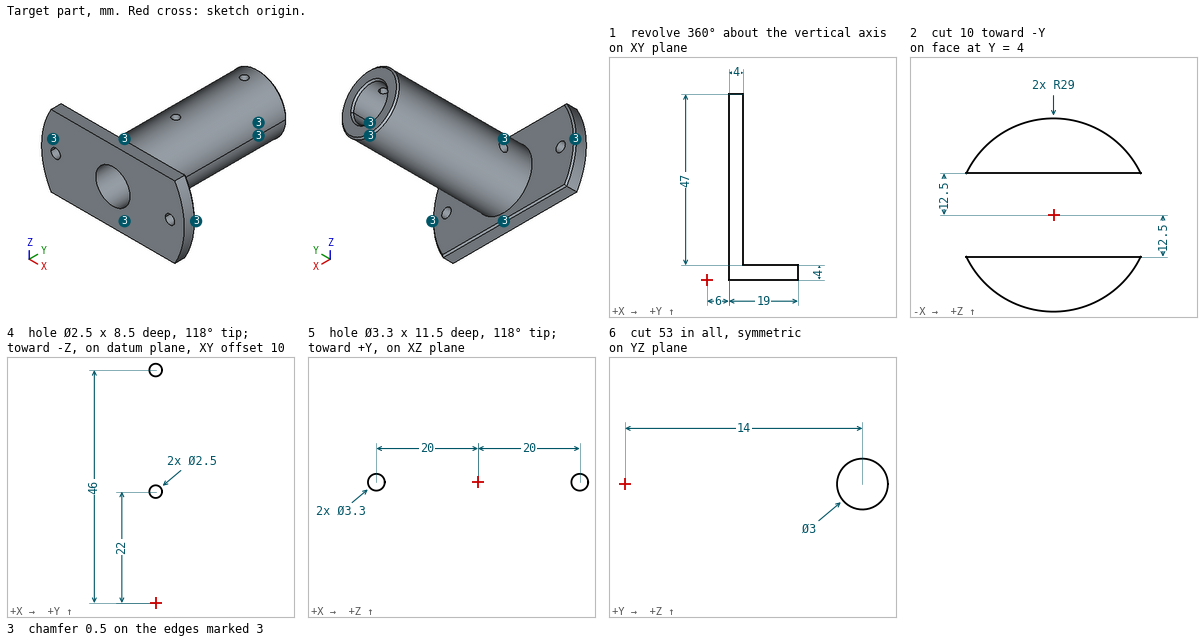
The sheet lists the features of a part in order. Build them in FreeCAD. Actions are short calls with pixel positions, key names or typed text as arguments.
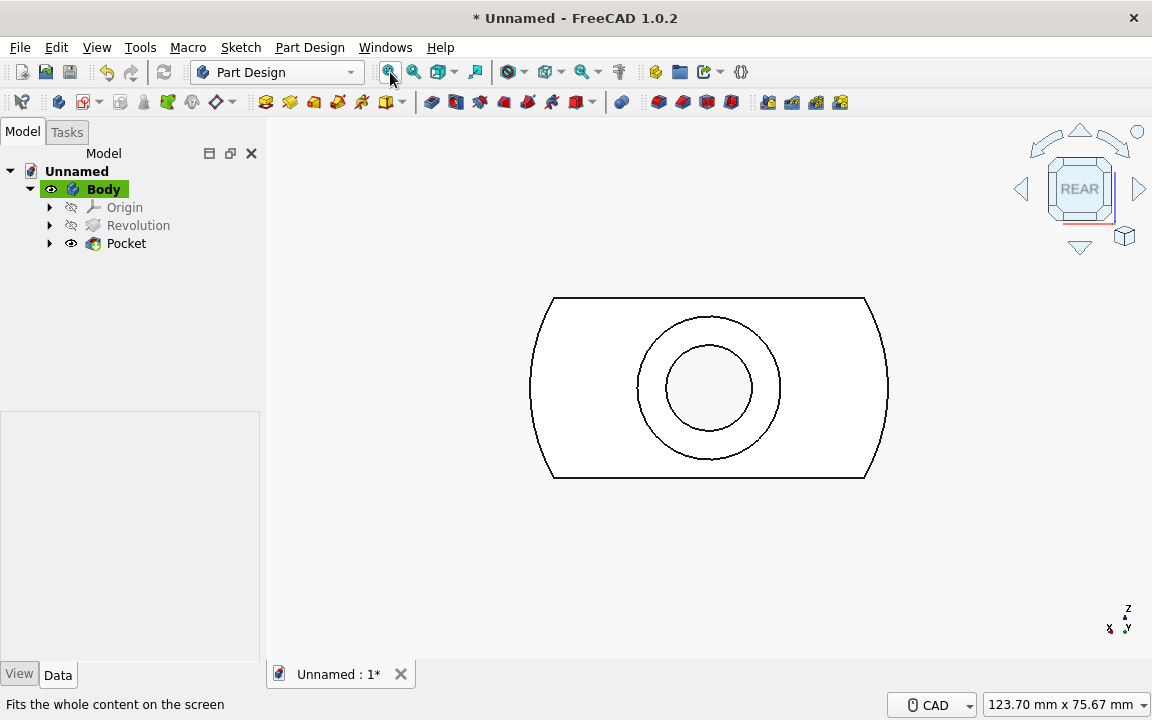
click(888, 387)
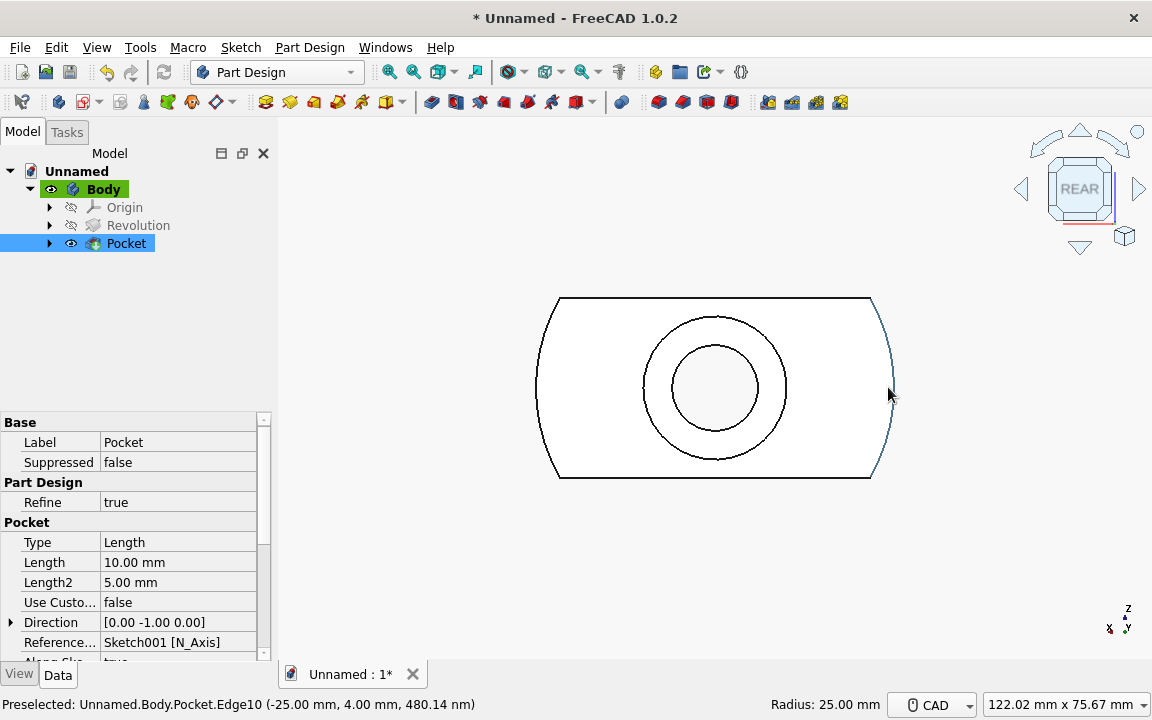
click(715, 477, ctrl)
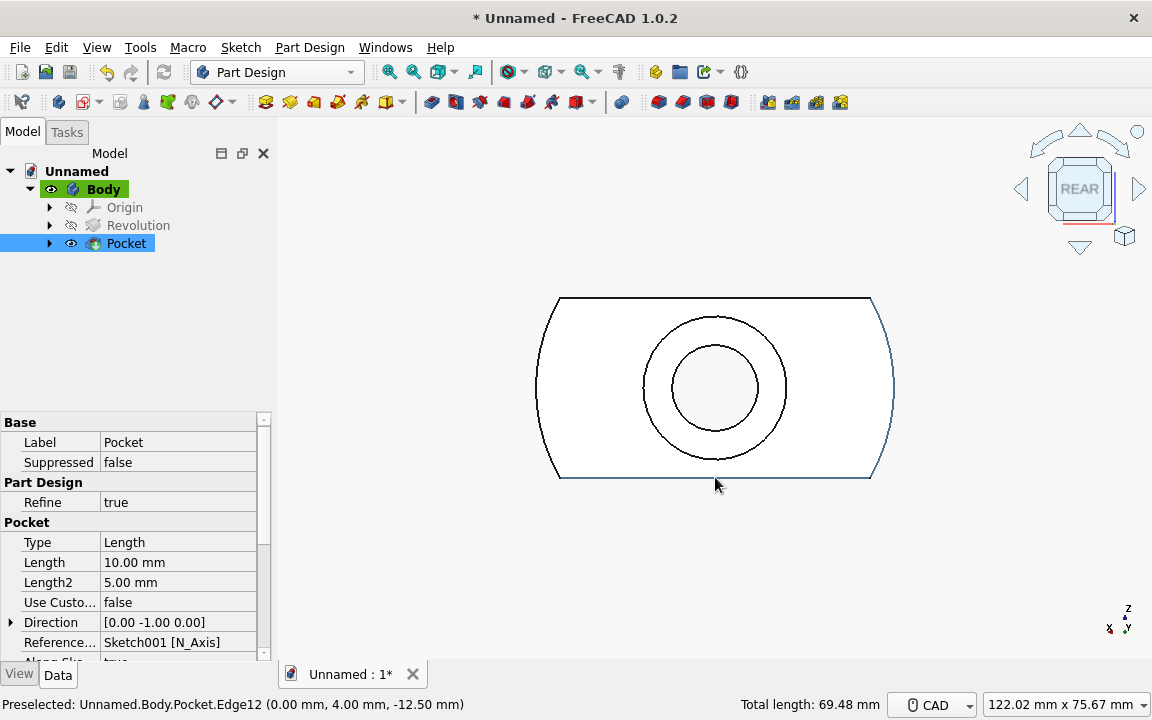
click(715, 297, ctrl)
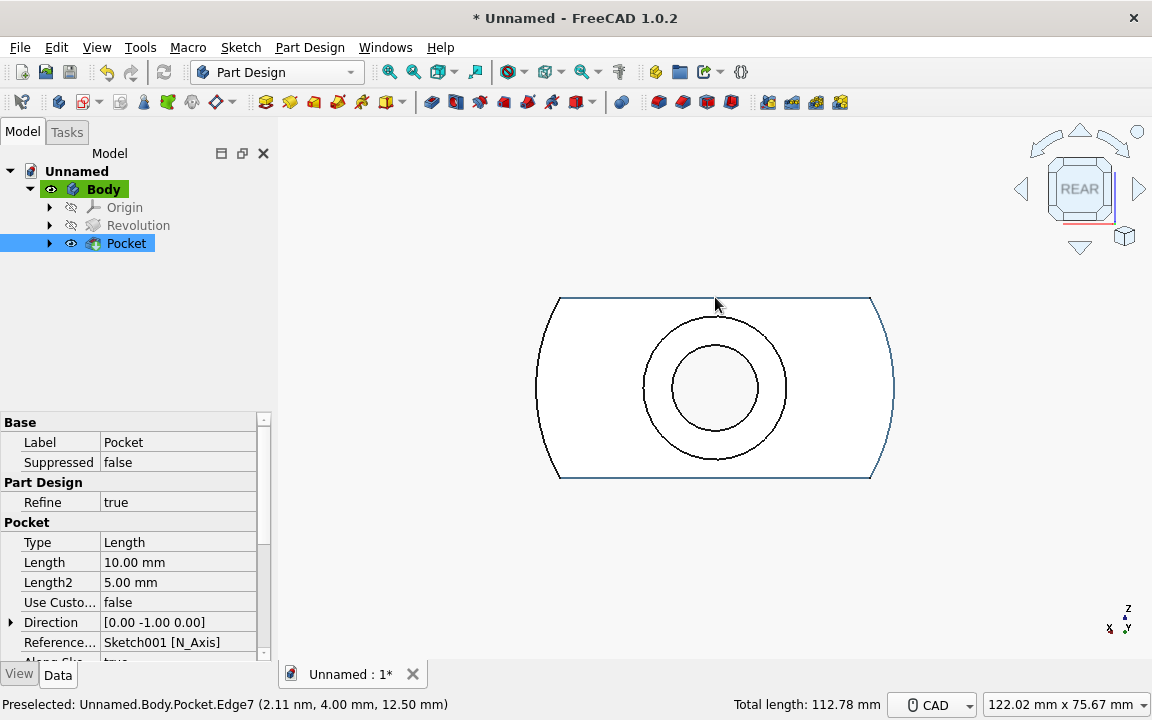
click(702, 346, ctrl)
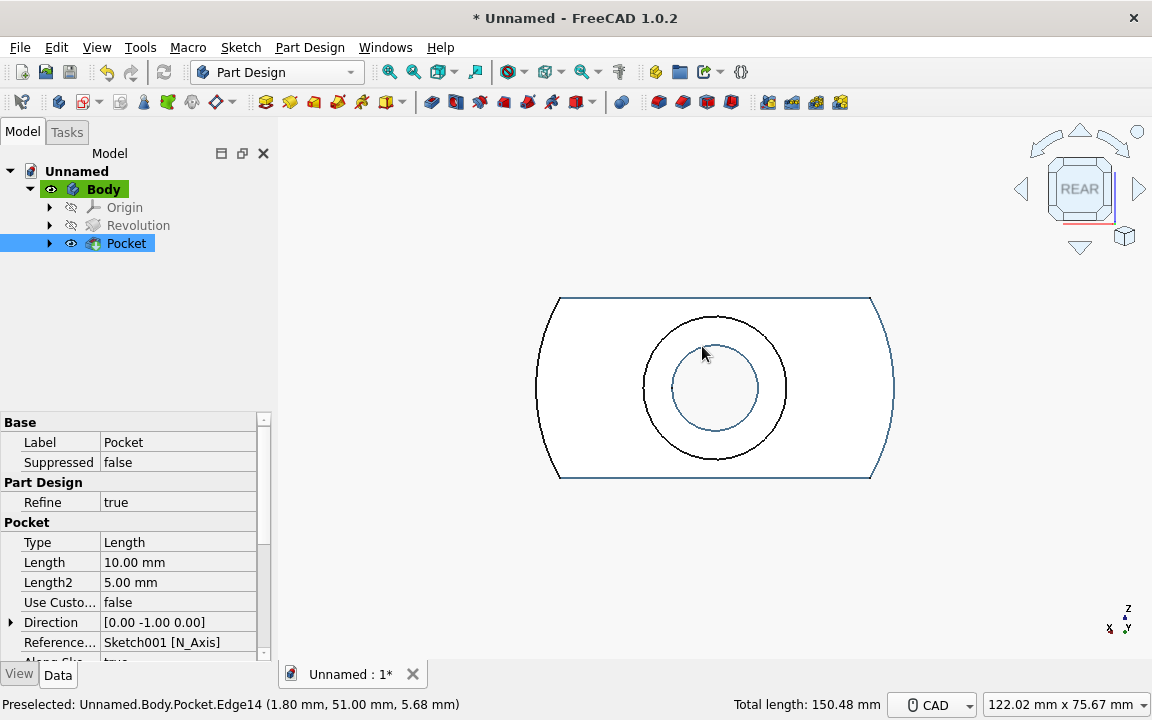
click(787, 387, ctrl)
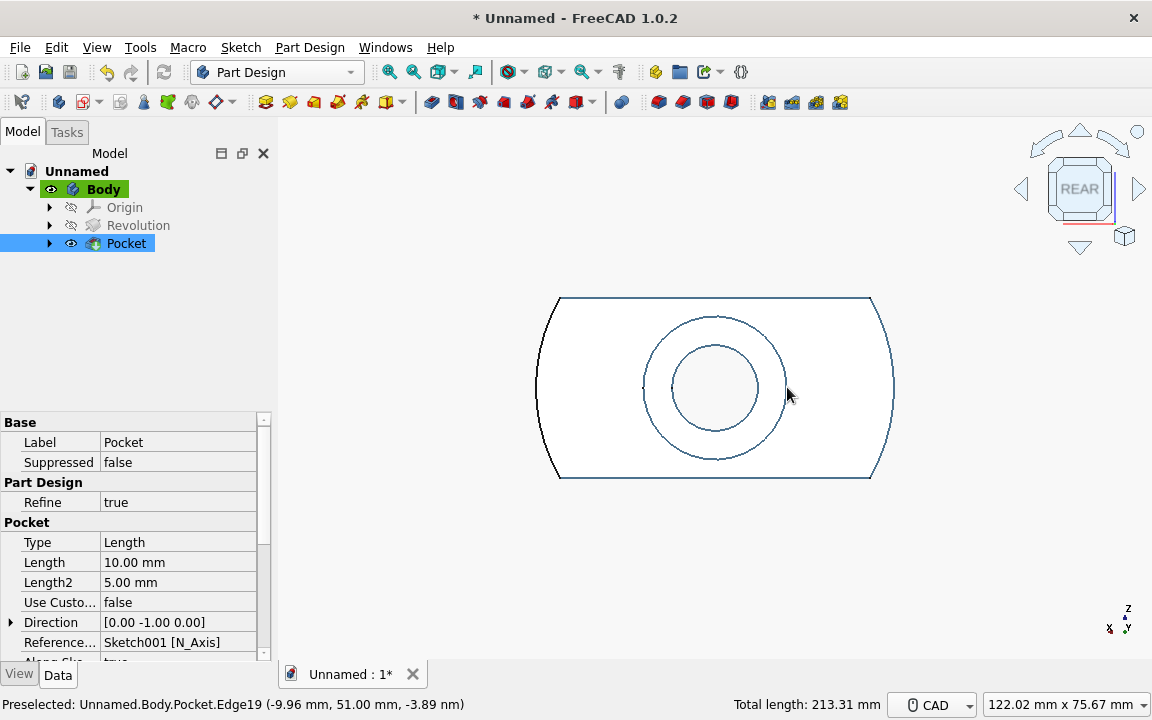
key(0)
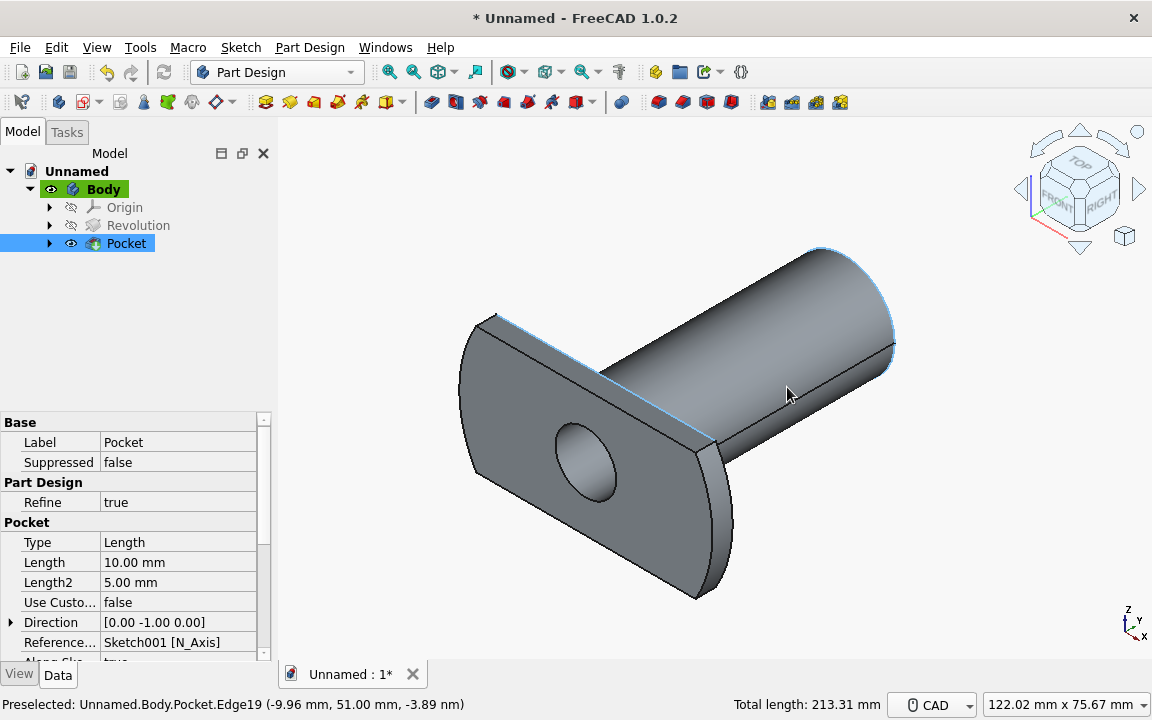
key(2)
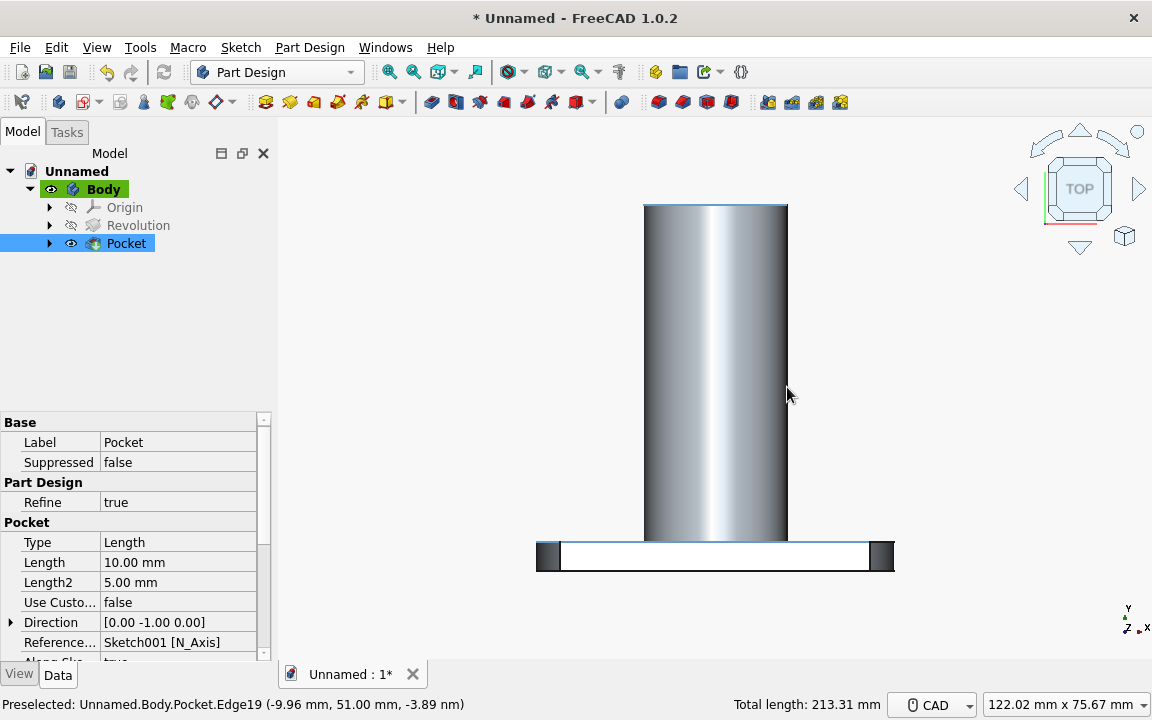
key(1)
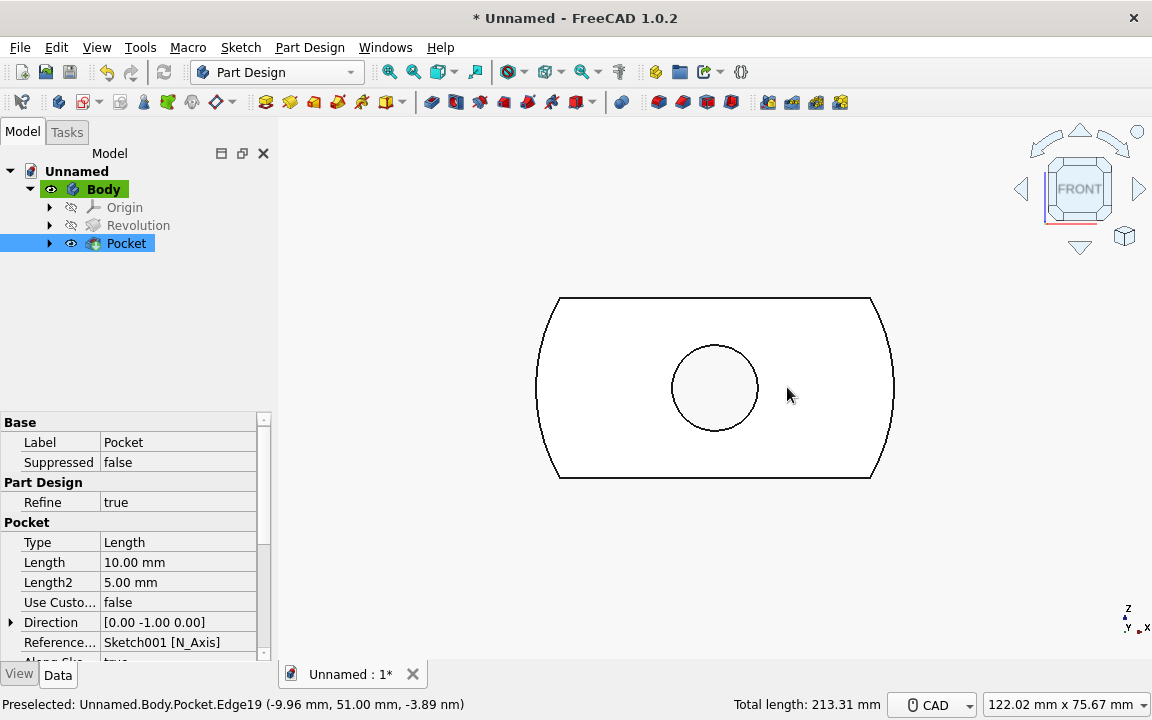
click(390, 72)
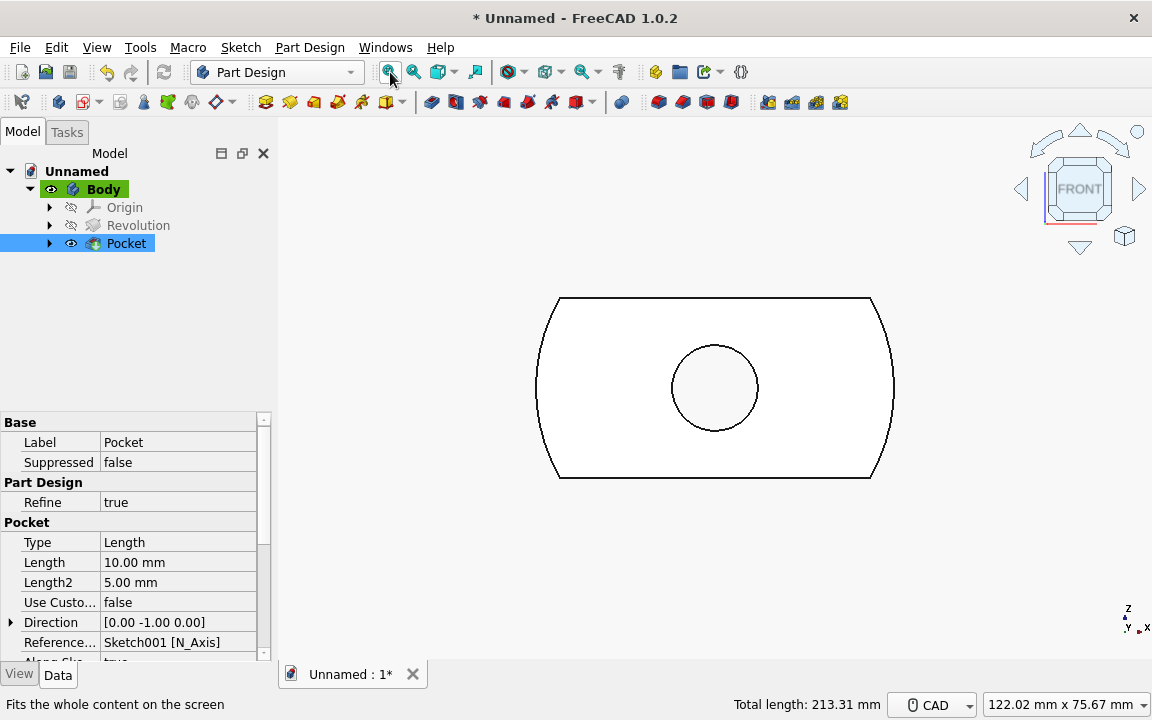
key(3)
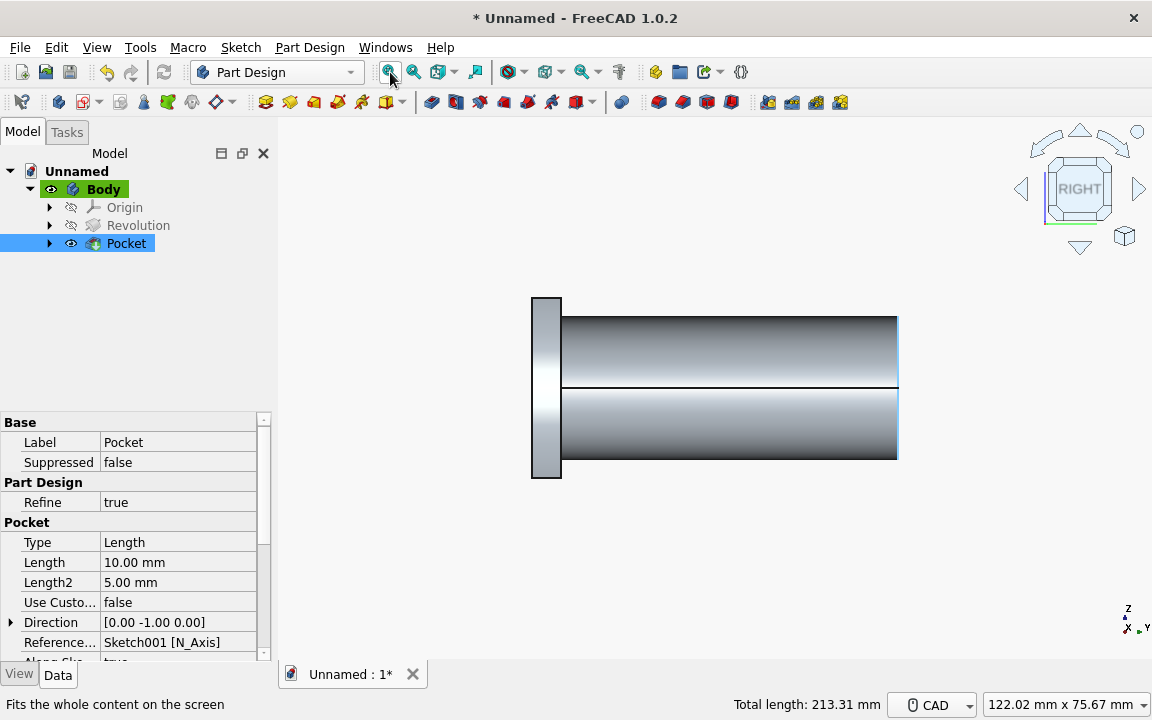
click(390, 72)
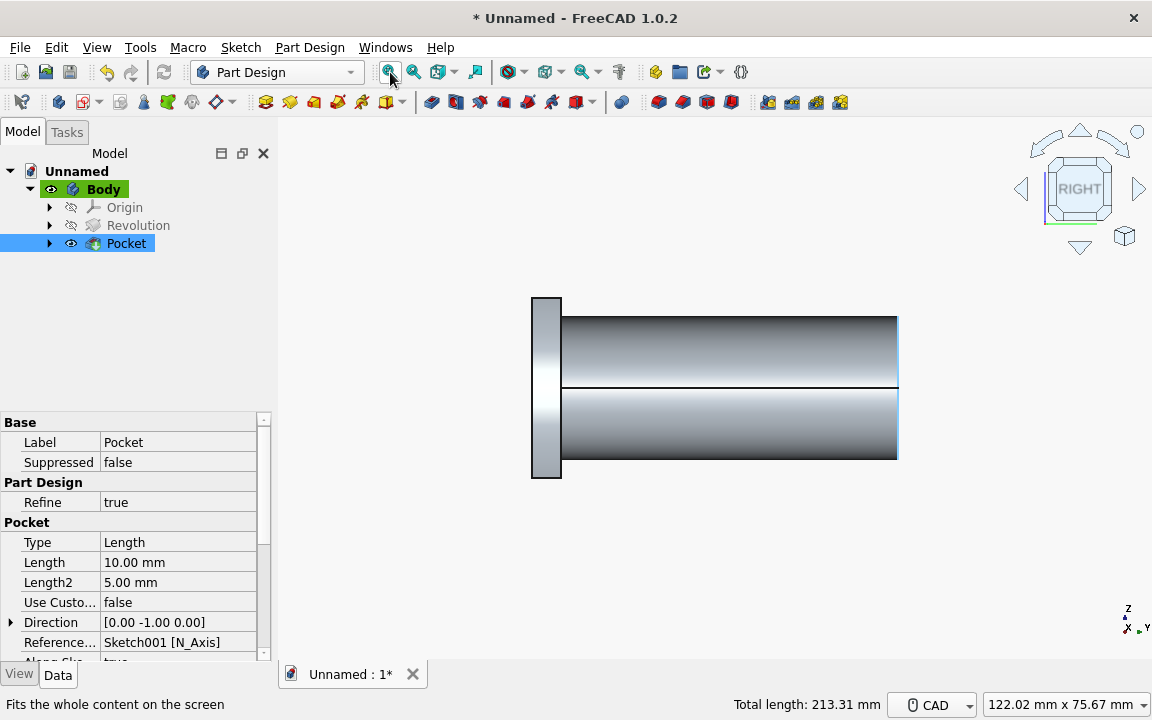
click(561, 433, ctrl)